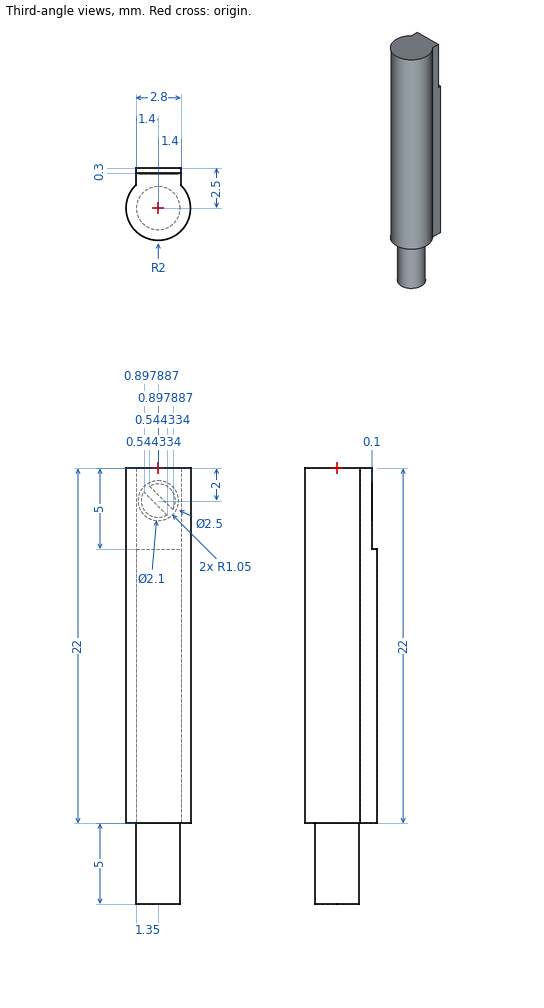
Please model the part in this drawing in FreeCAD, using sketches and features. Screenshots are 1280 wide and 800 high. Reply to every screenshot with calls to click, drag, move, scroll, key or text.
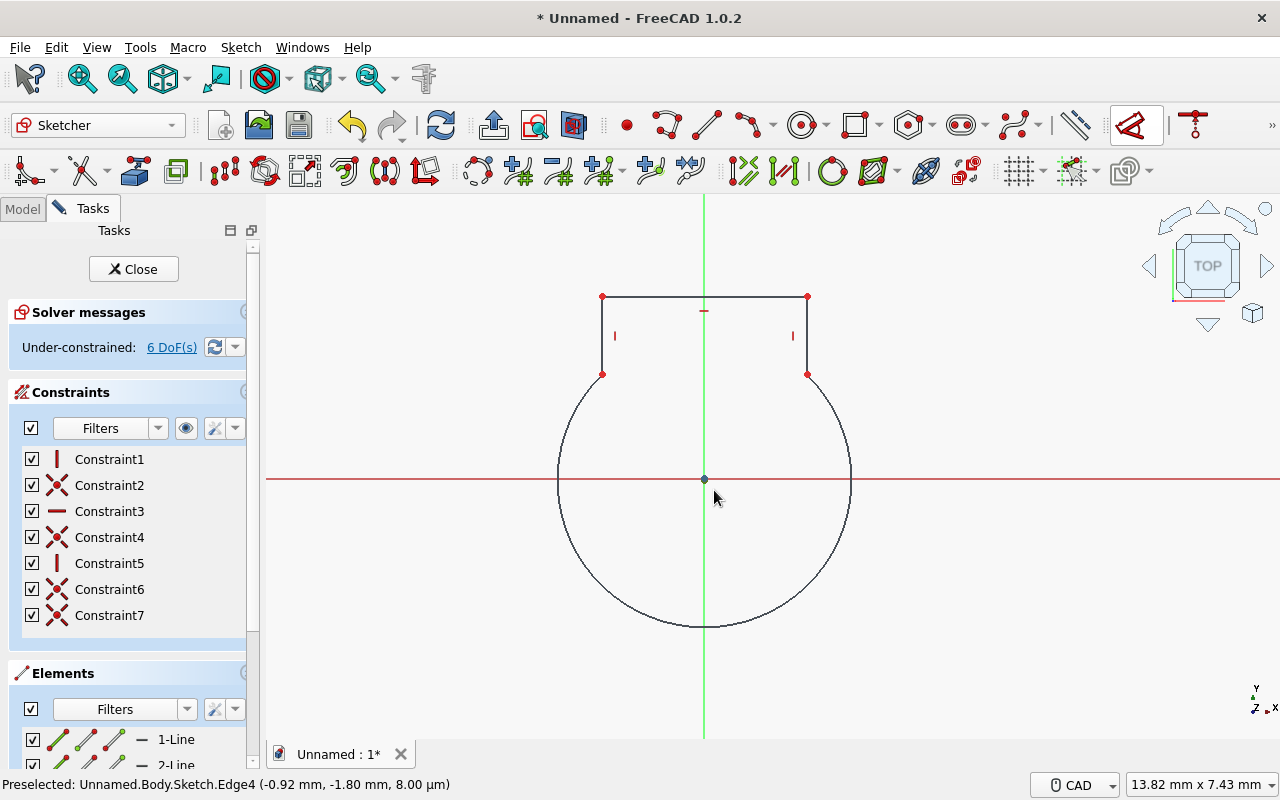
click(1194, 126)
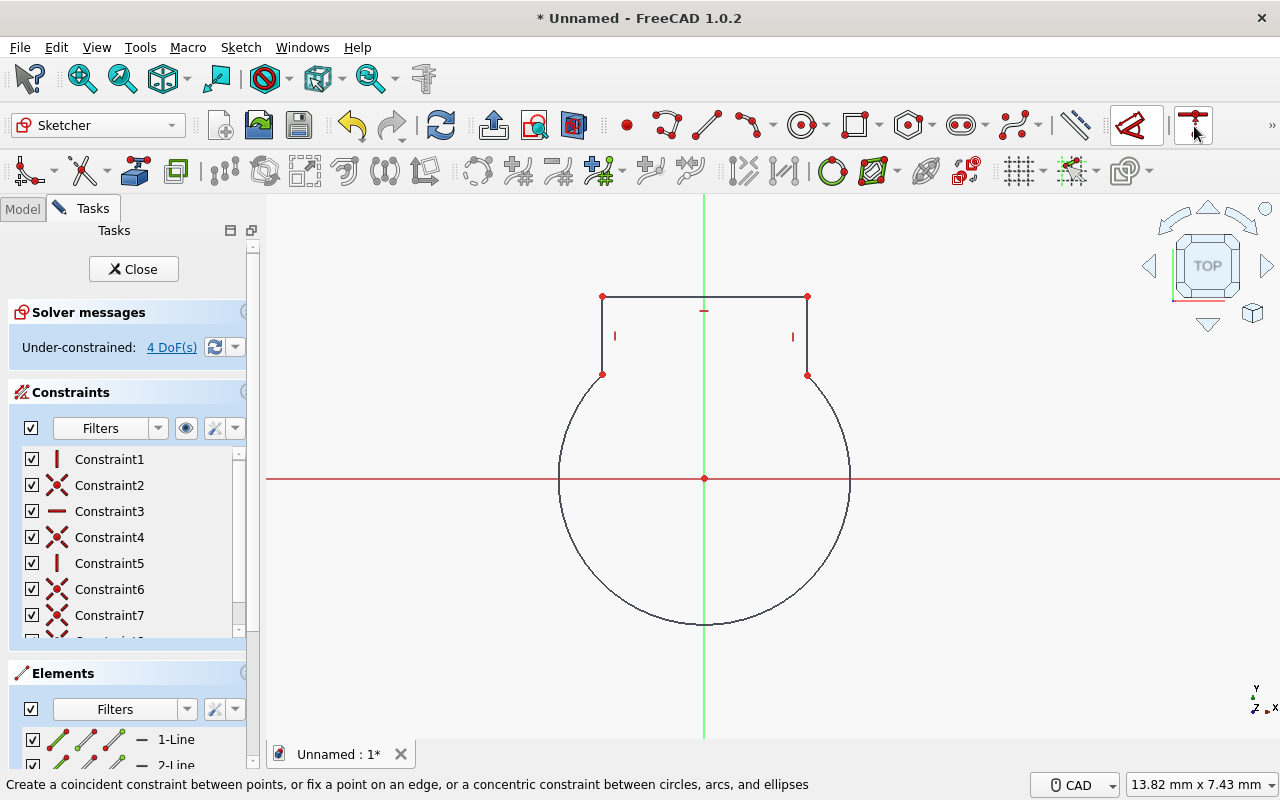
click(1130, 126)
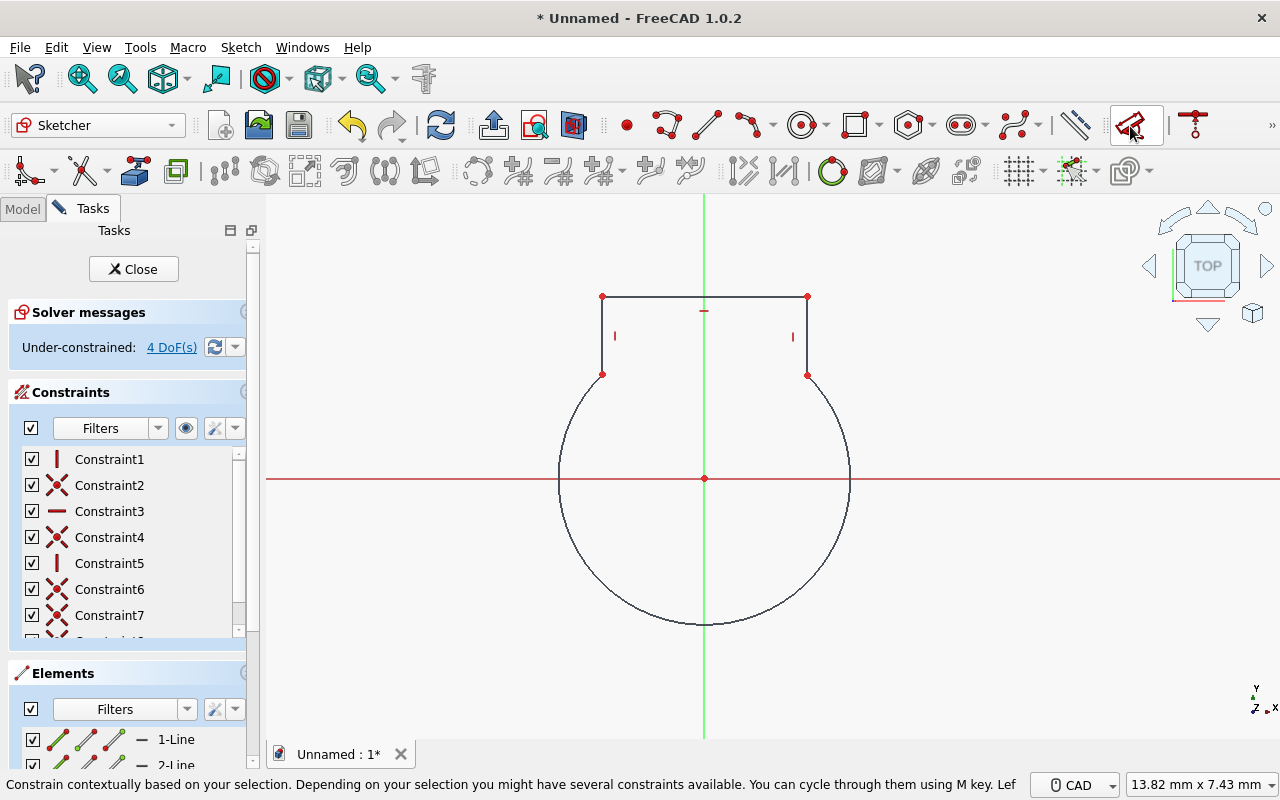
click(586, 564)
click(560, 583)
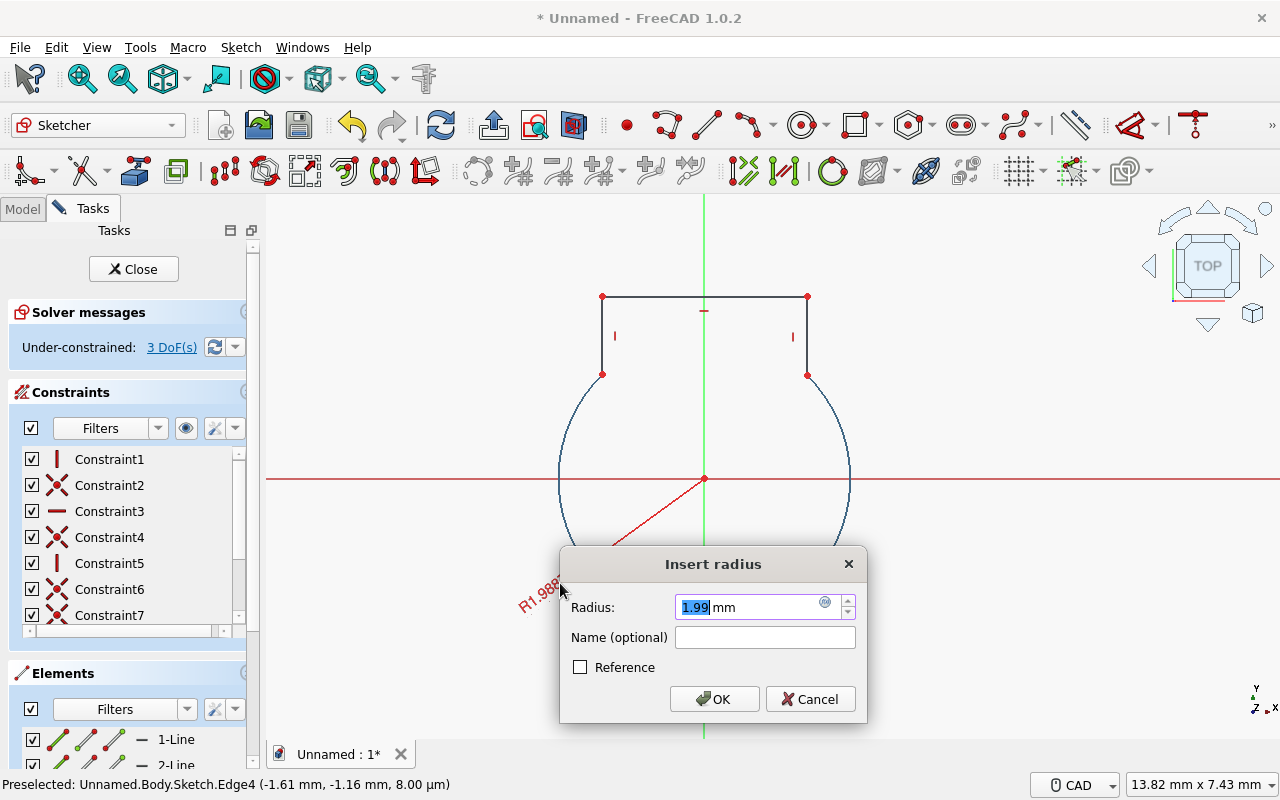
text(2)
key(Return)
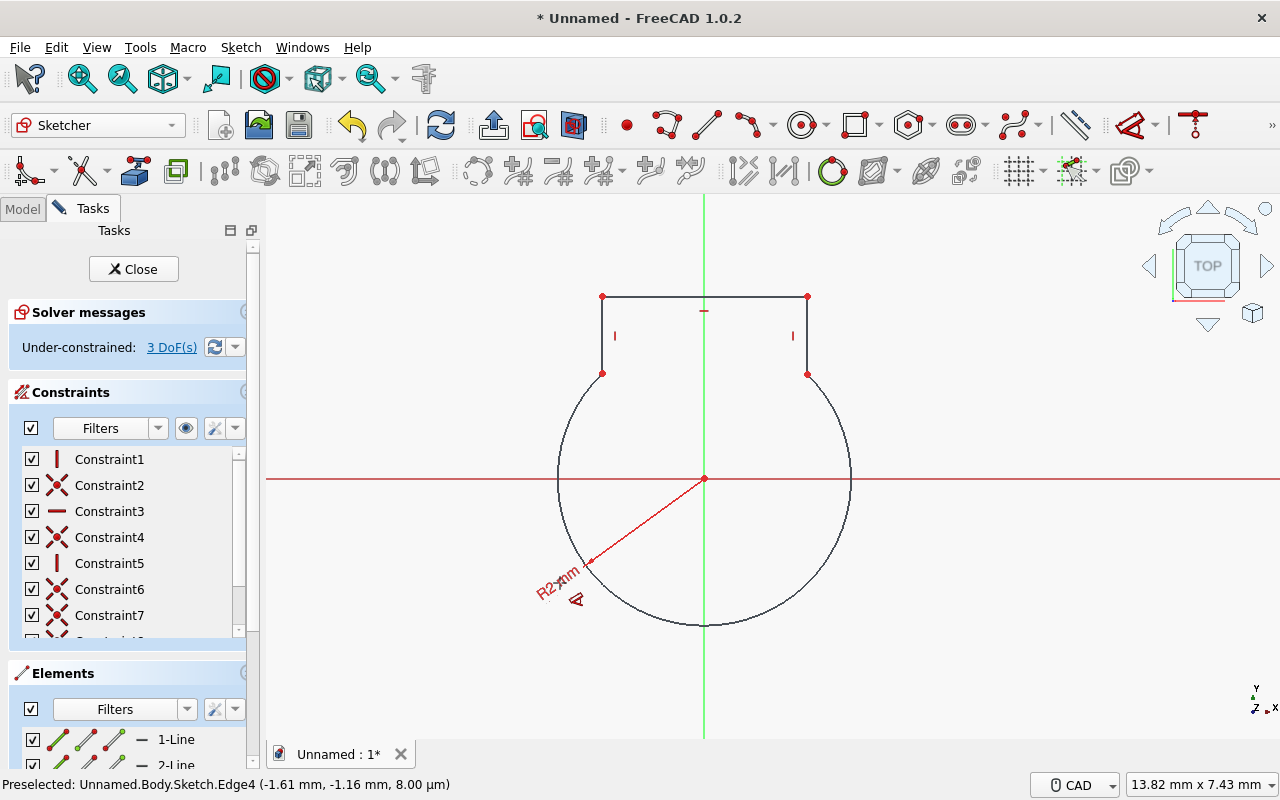
click(746, 297)
click(657, 263)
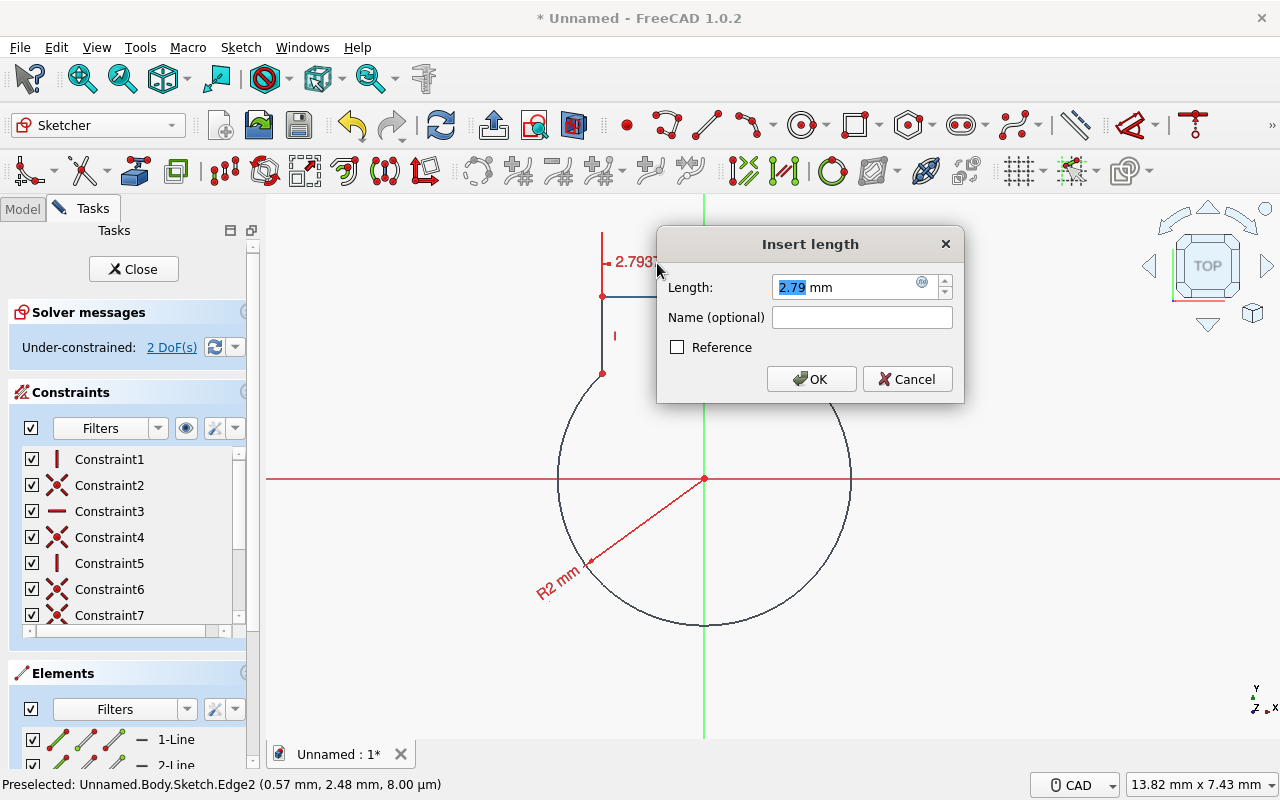
text(2.8)
key(Return)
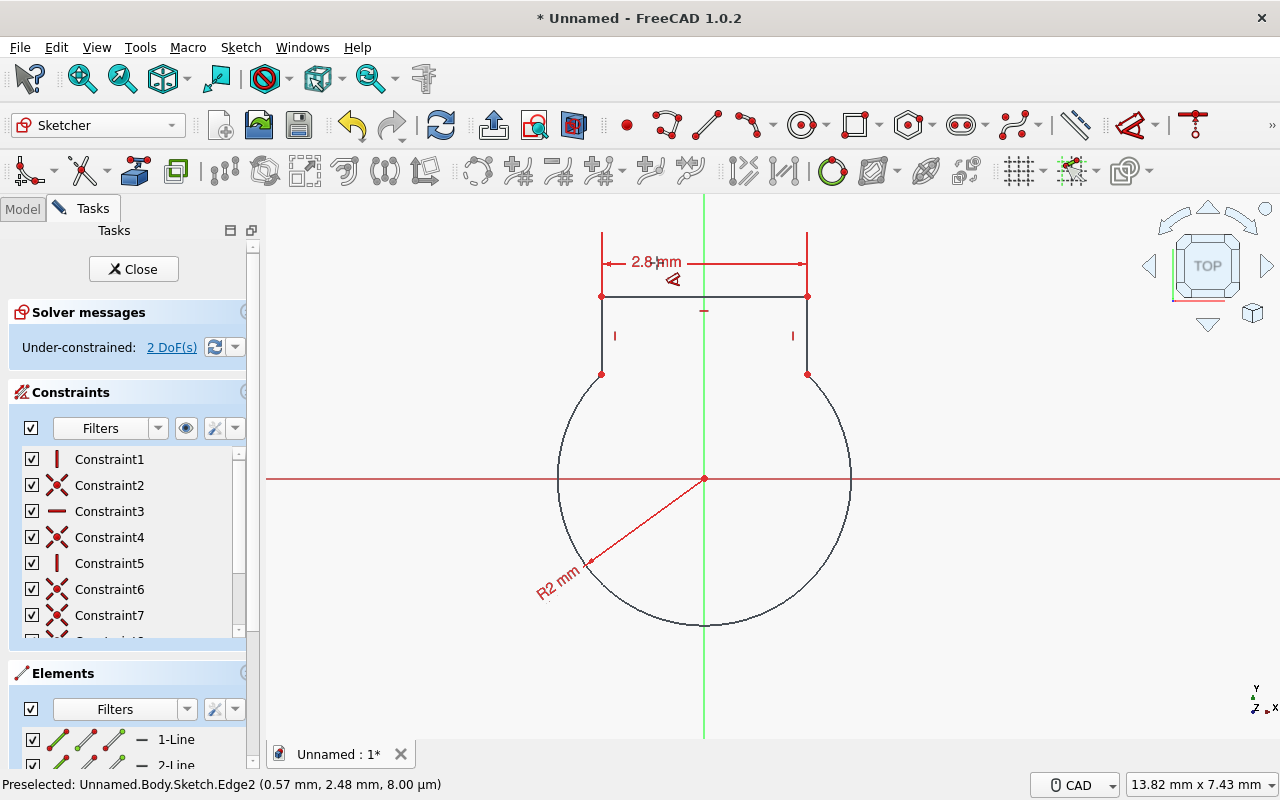
click(807, 374)
click(756, 340)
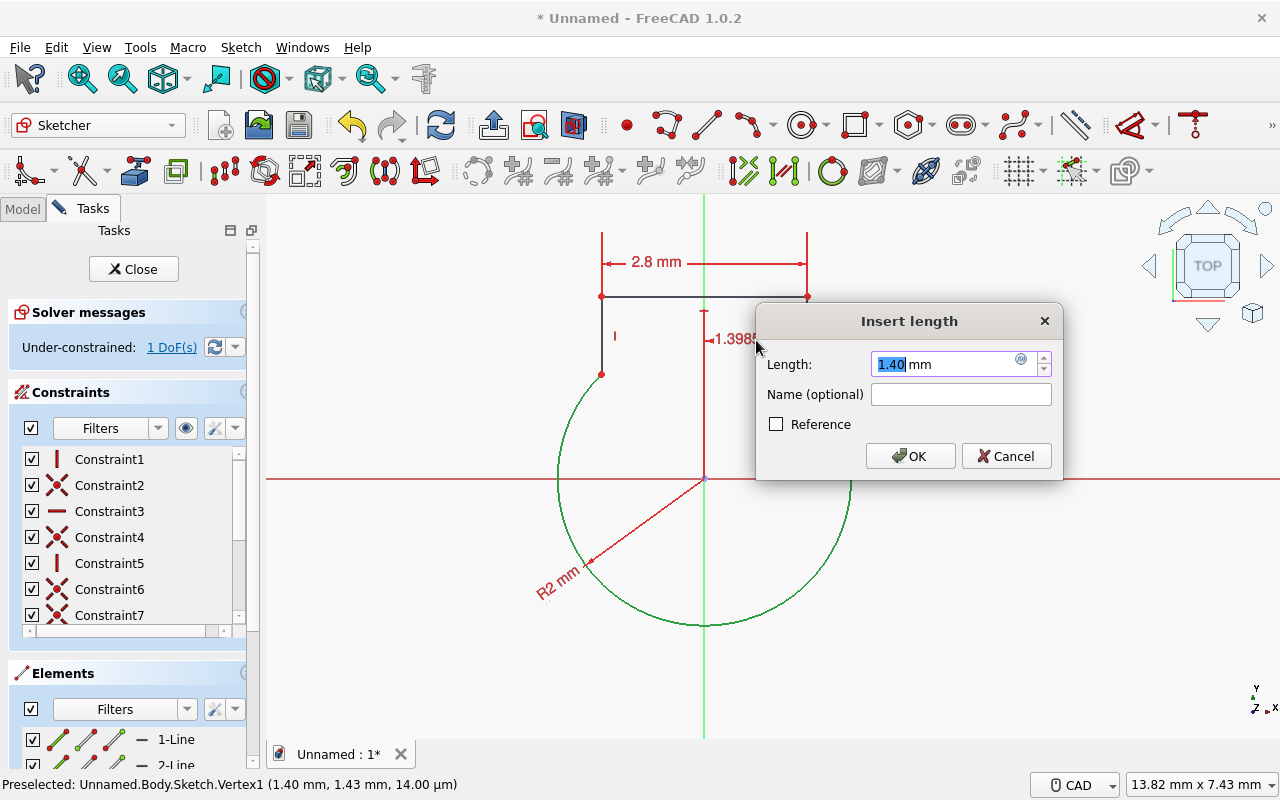
text(1.4)
key(Return)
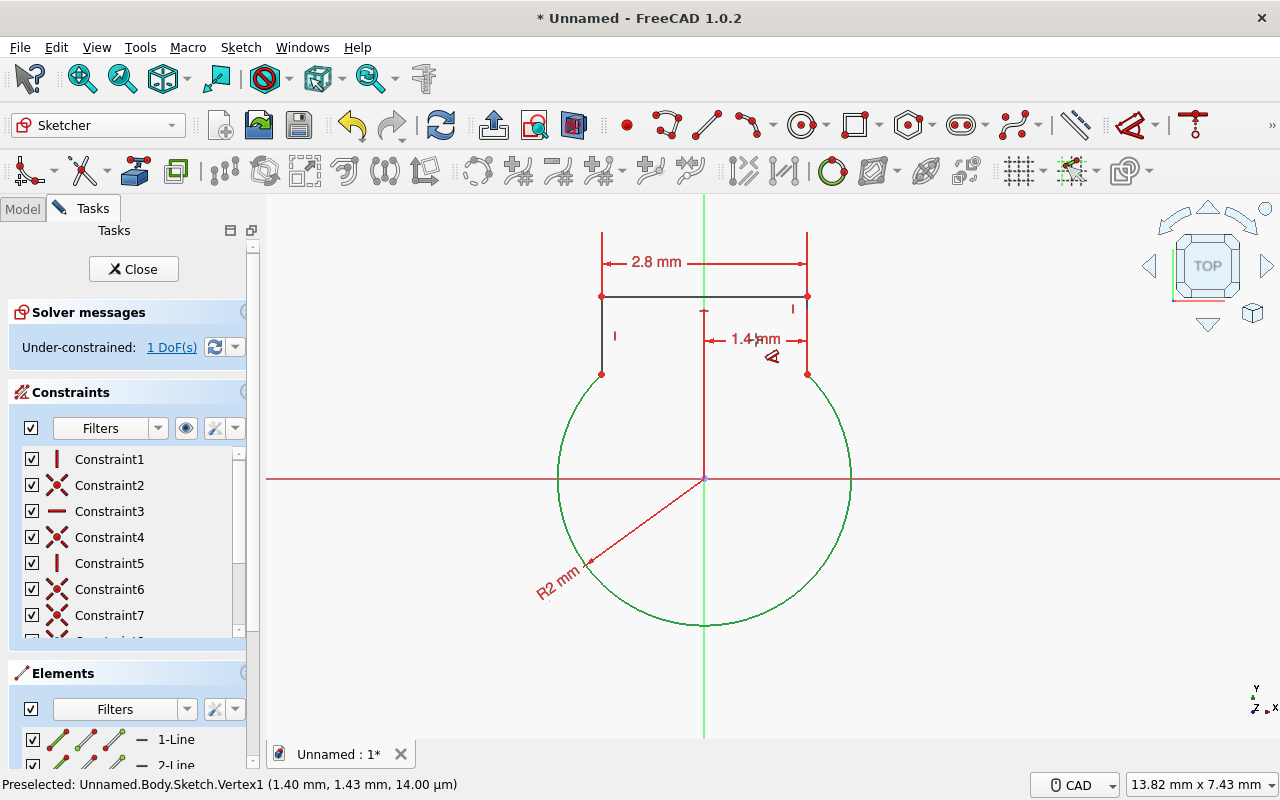
click(807, 297)
click(841, 388)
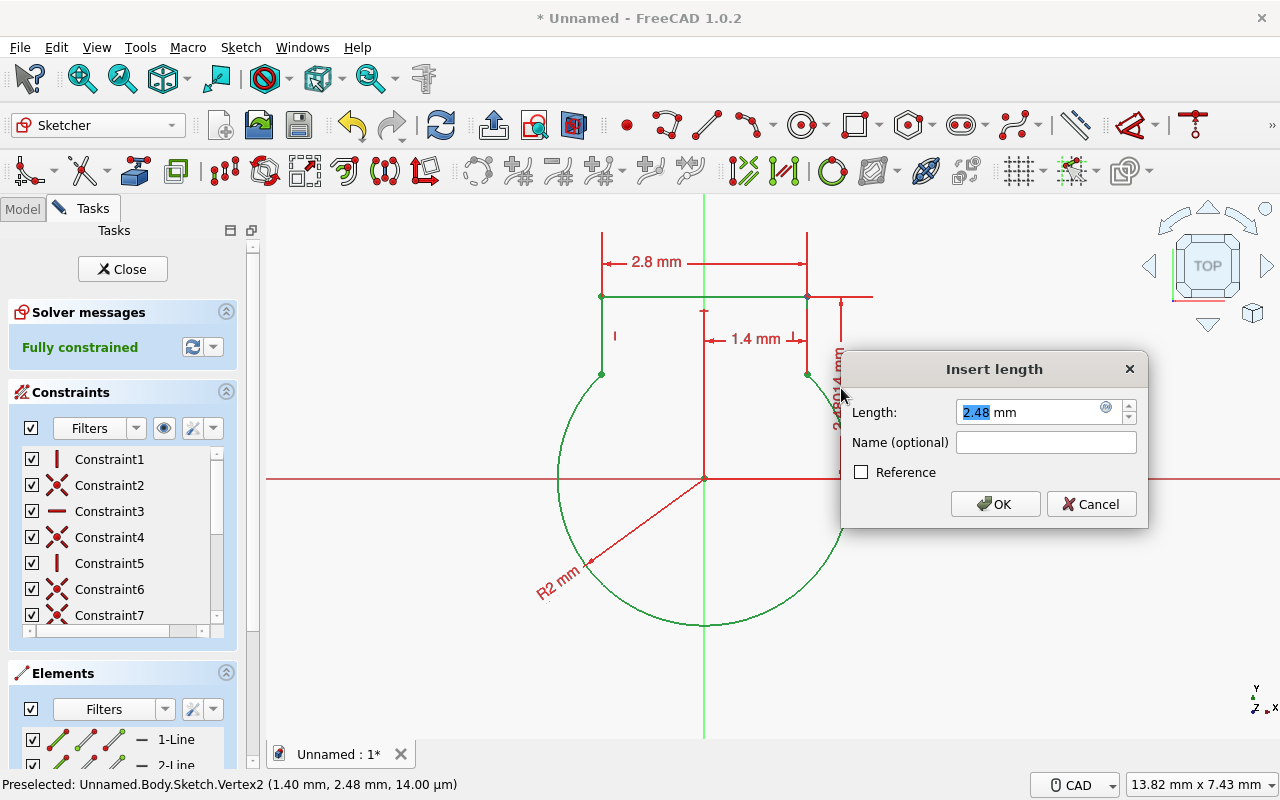
text(2.5)
key(Return)
key(Escape)